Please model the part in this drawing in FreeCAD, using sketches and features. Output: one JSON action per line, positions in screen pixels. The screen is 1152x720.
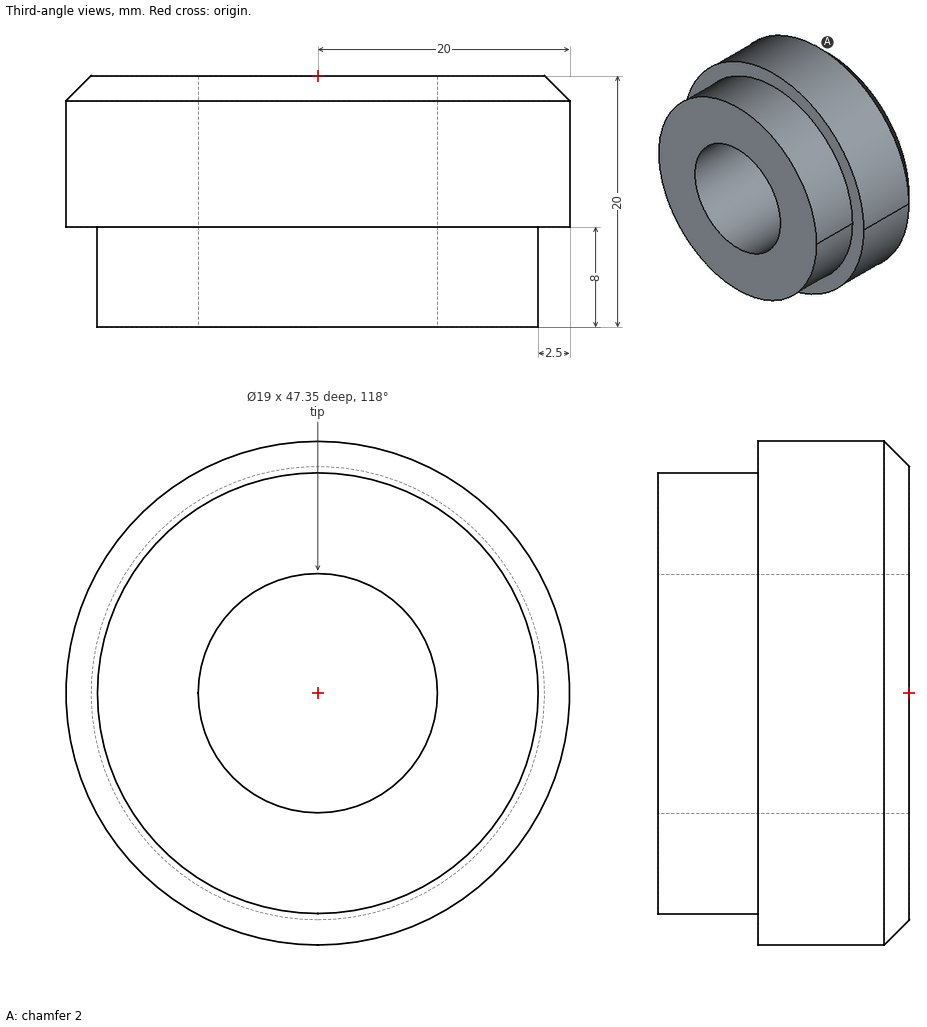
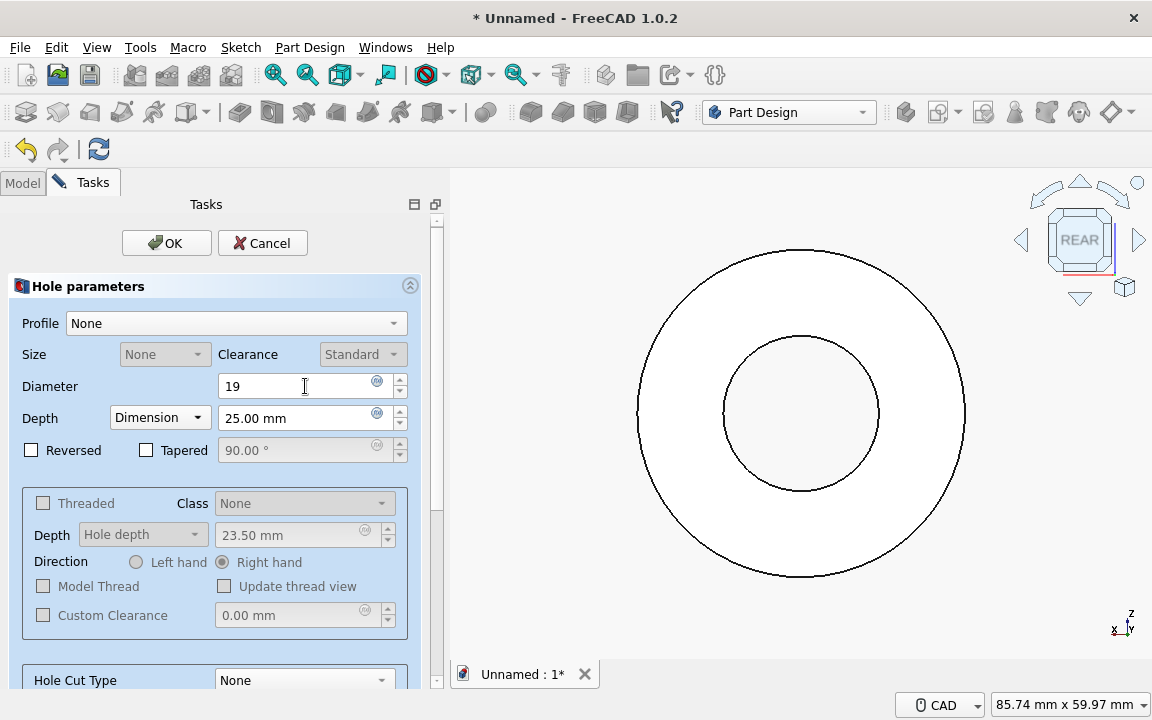
{"action": "triple_click", "coordinate": [305, 418]}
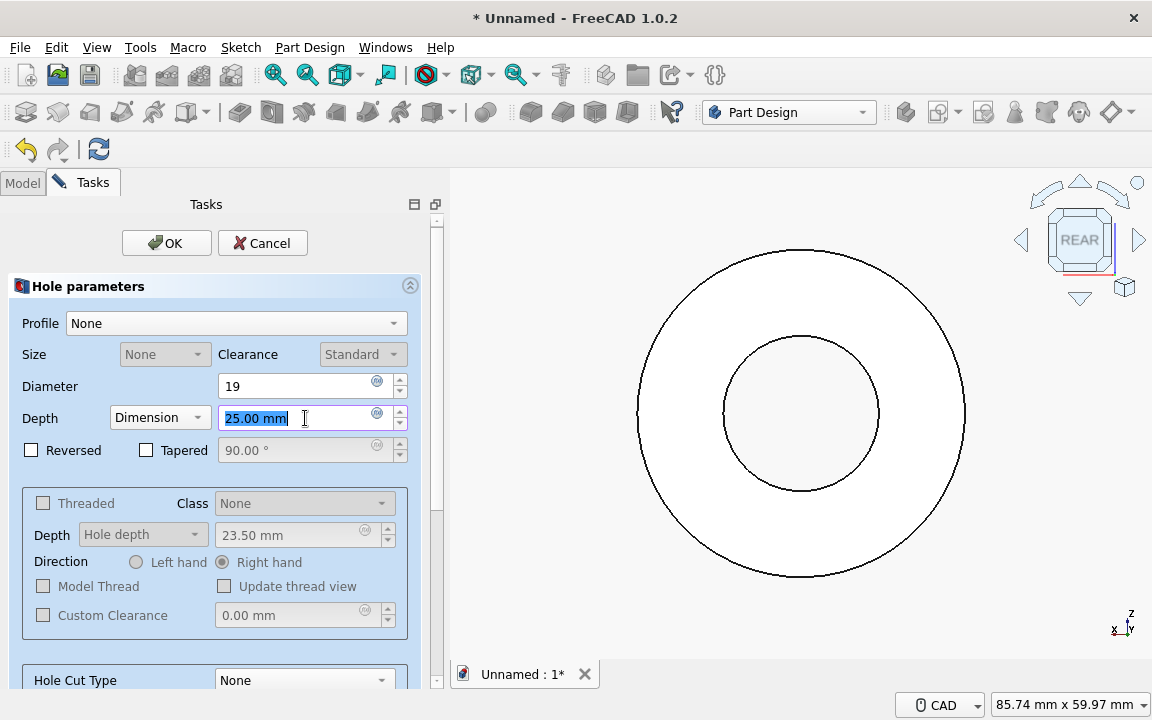
{"action": "type", "text": "47.35"}
{"action": "key", "text": "Tab"}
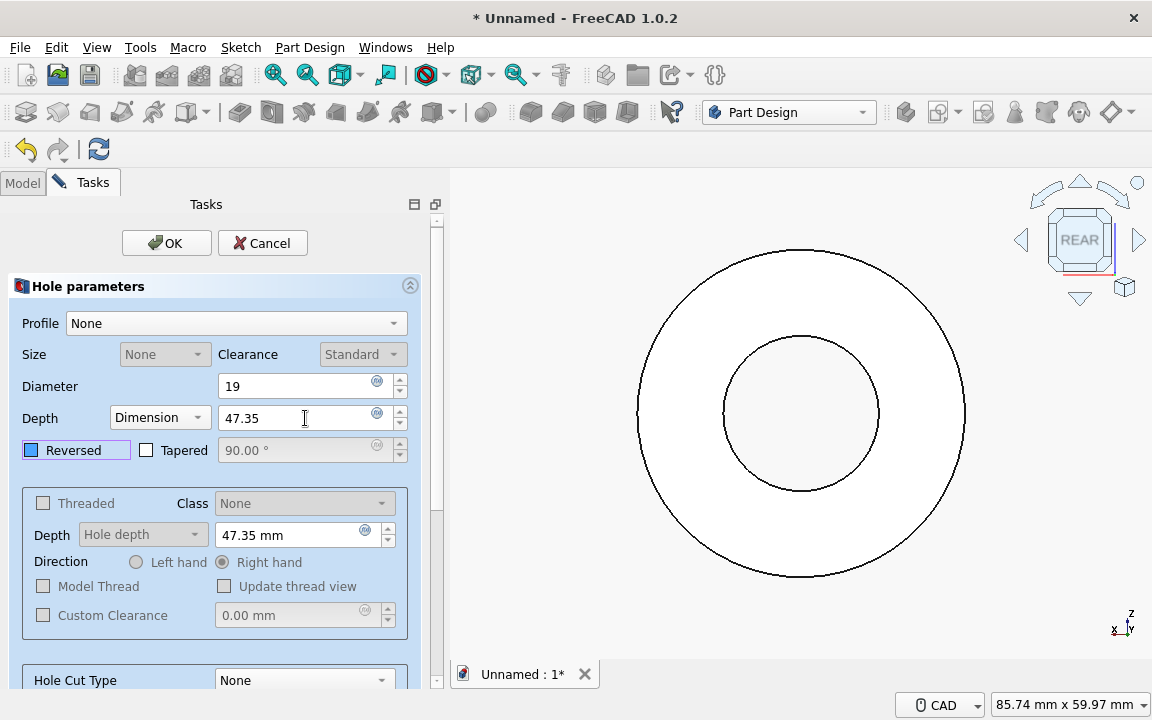
{"action": "left_click", "coordinate": [167, 243]}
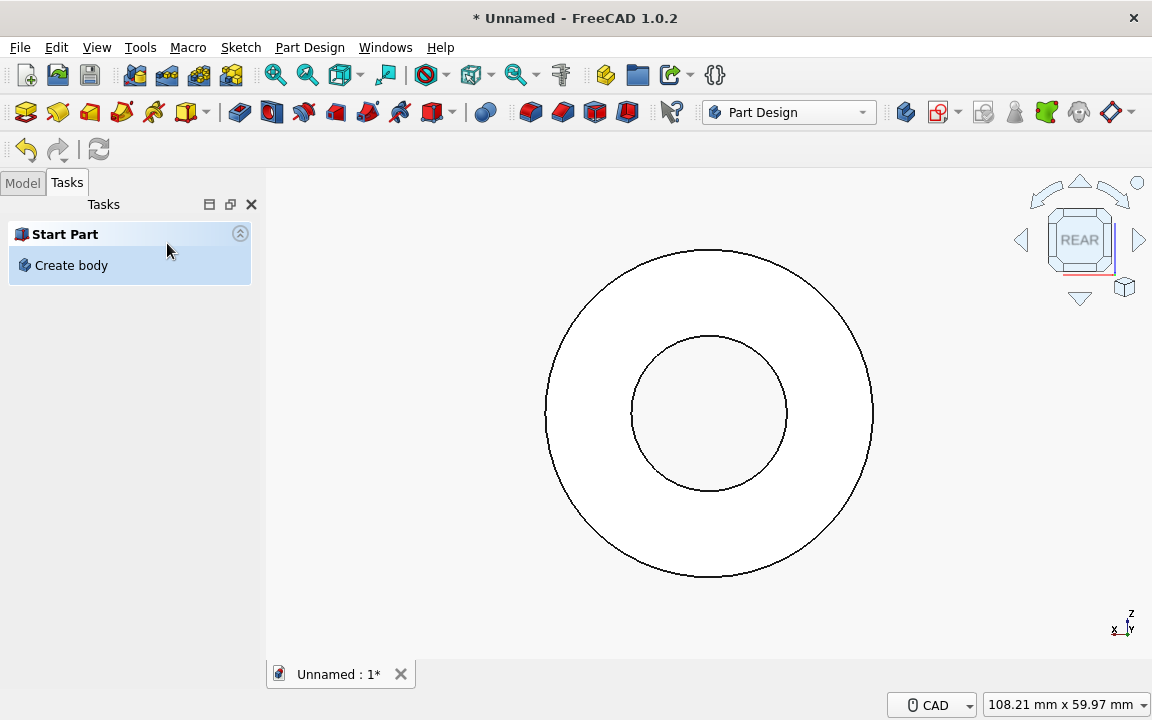
{"action": "left_click", "coordinate": [873, 413]}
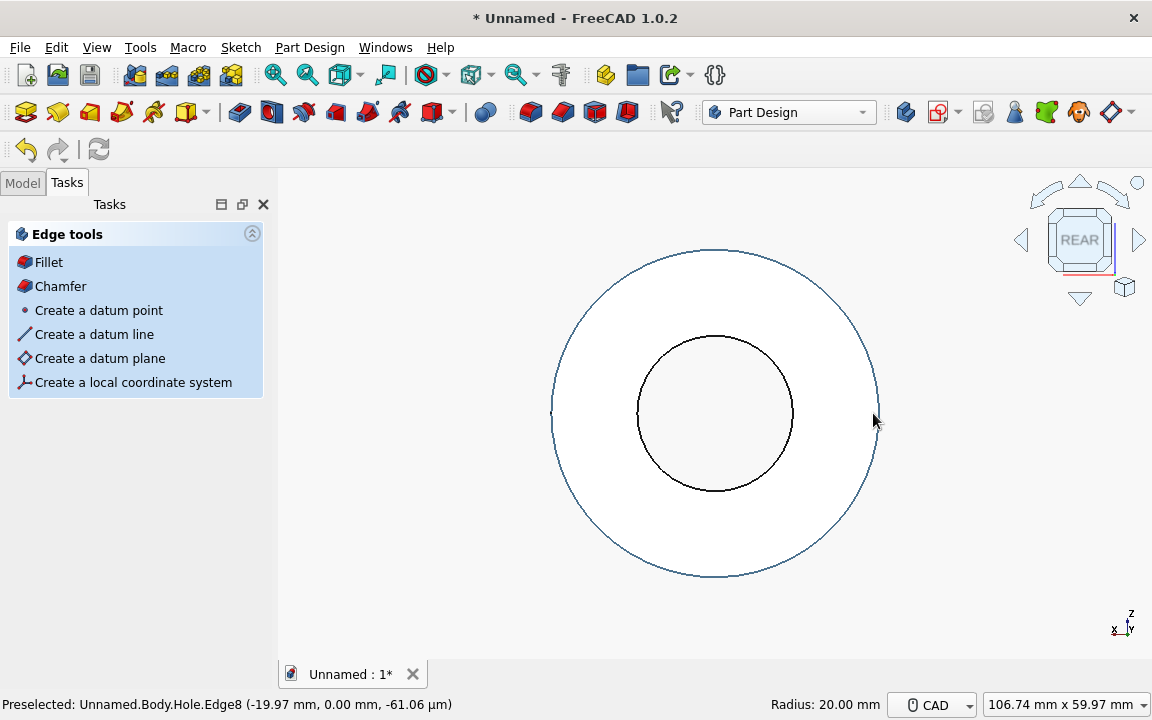
{"action": "left_click", "coordinate": [564, 112]}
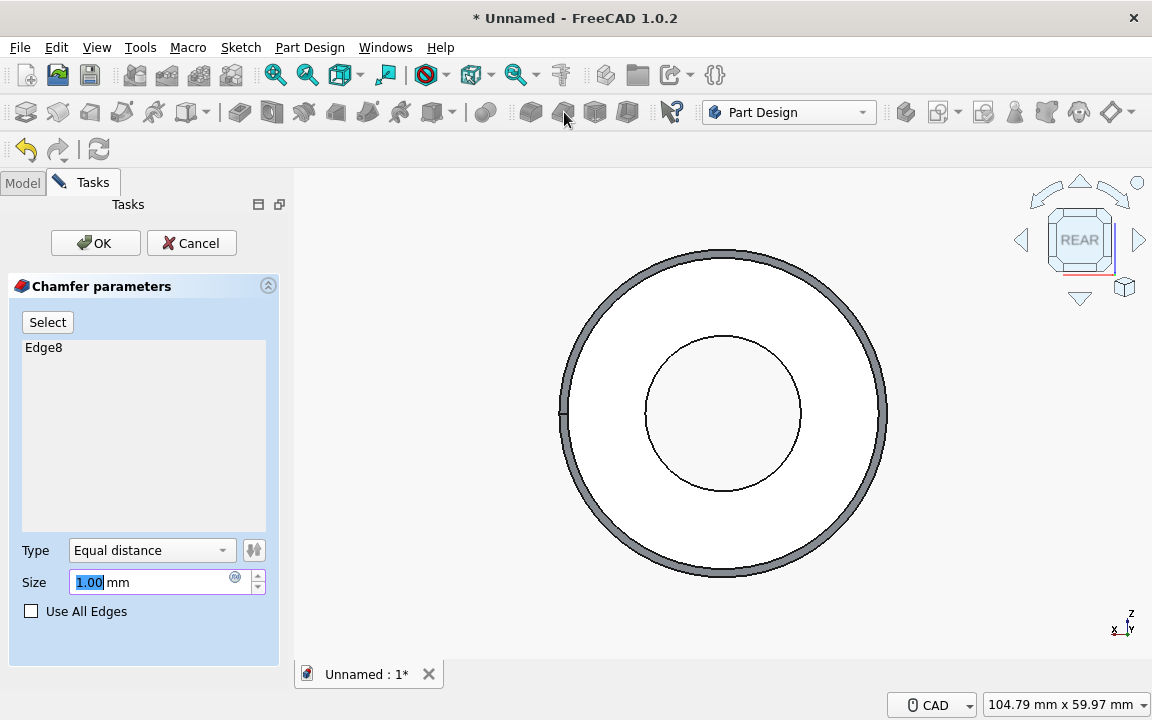
{"action": "type", "text": "2"}
{"action": "key", "text": "Tab"}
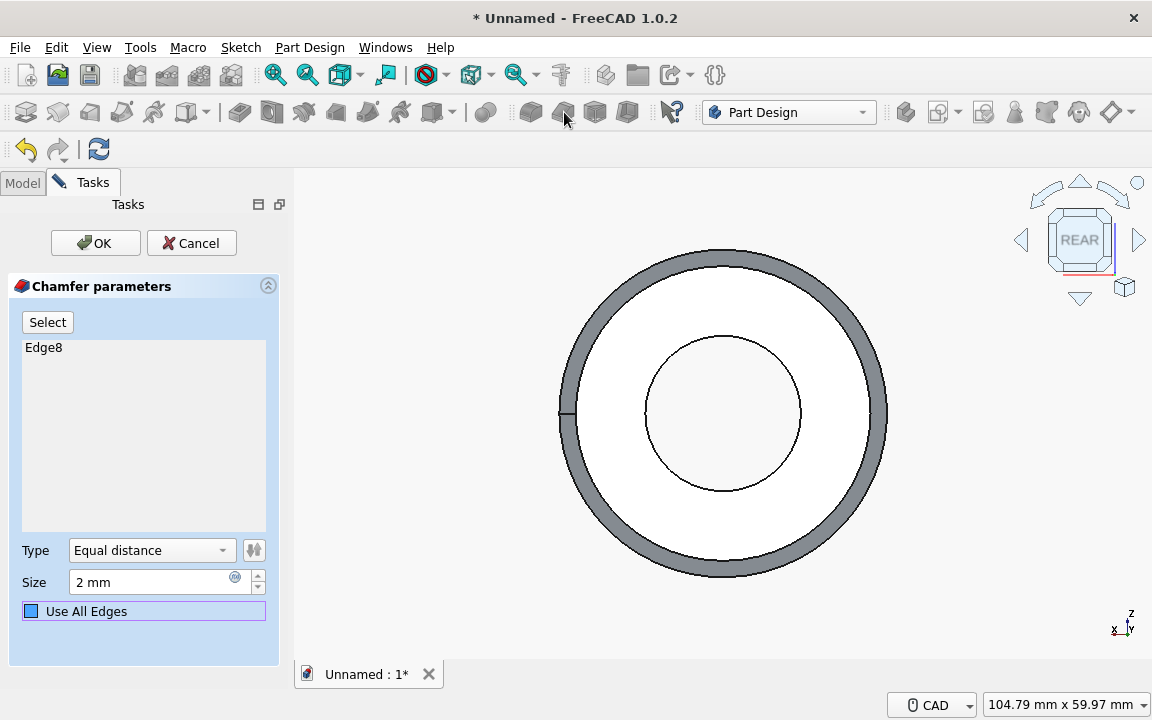
{"action": "left_click", "coordinate": [96, 243]}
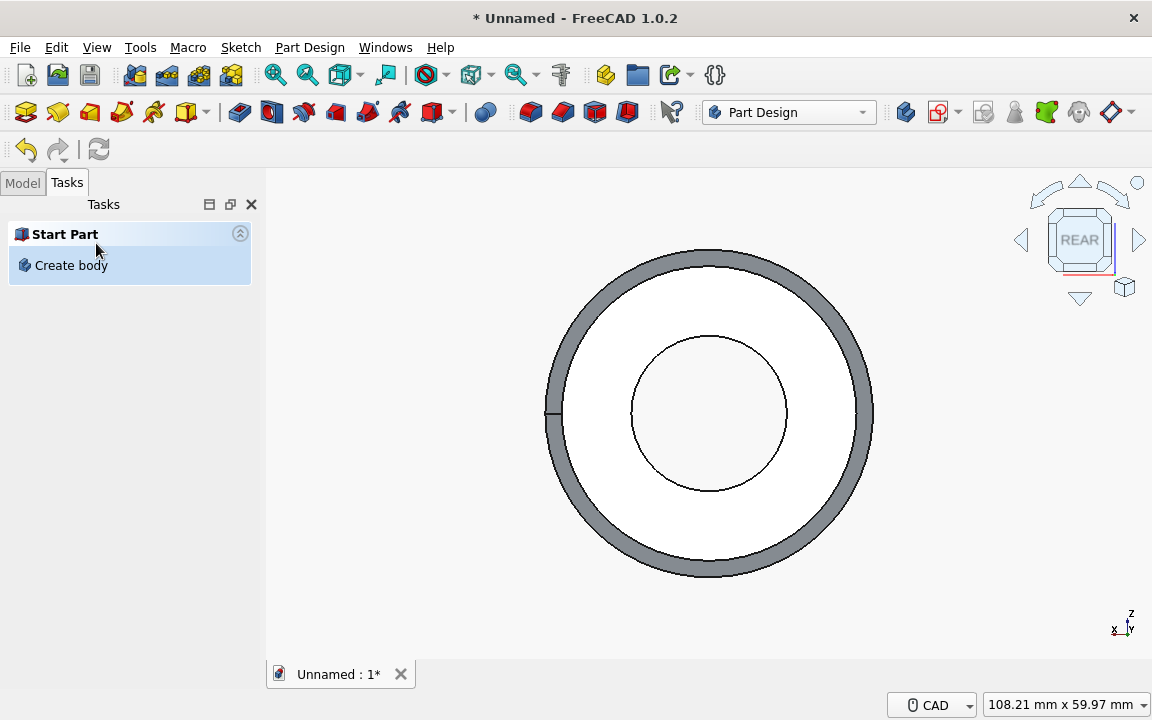
{"action": "key", "text": "0"}